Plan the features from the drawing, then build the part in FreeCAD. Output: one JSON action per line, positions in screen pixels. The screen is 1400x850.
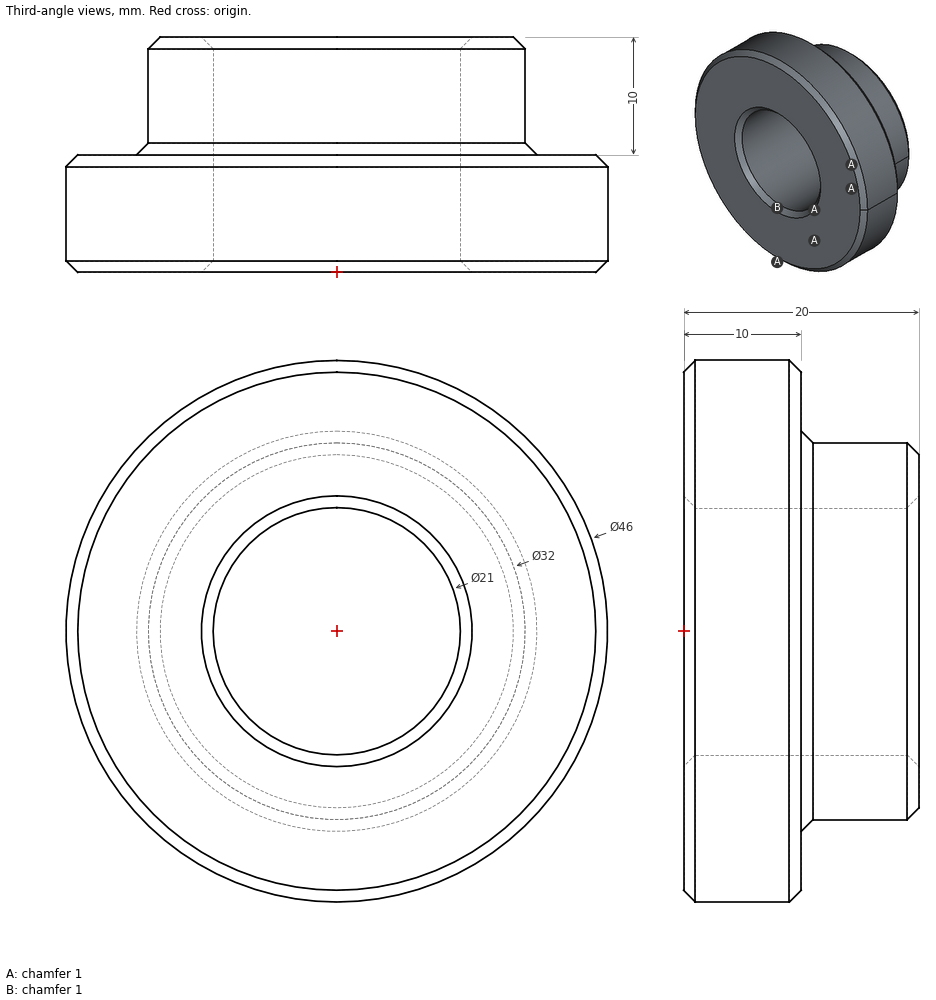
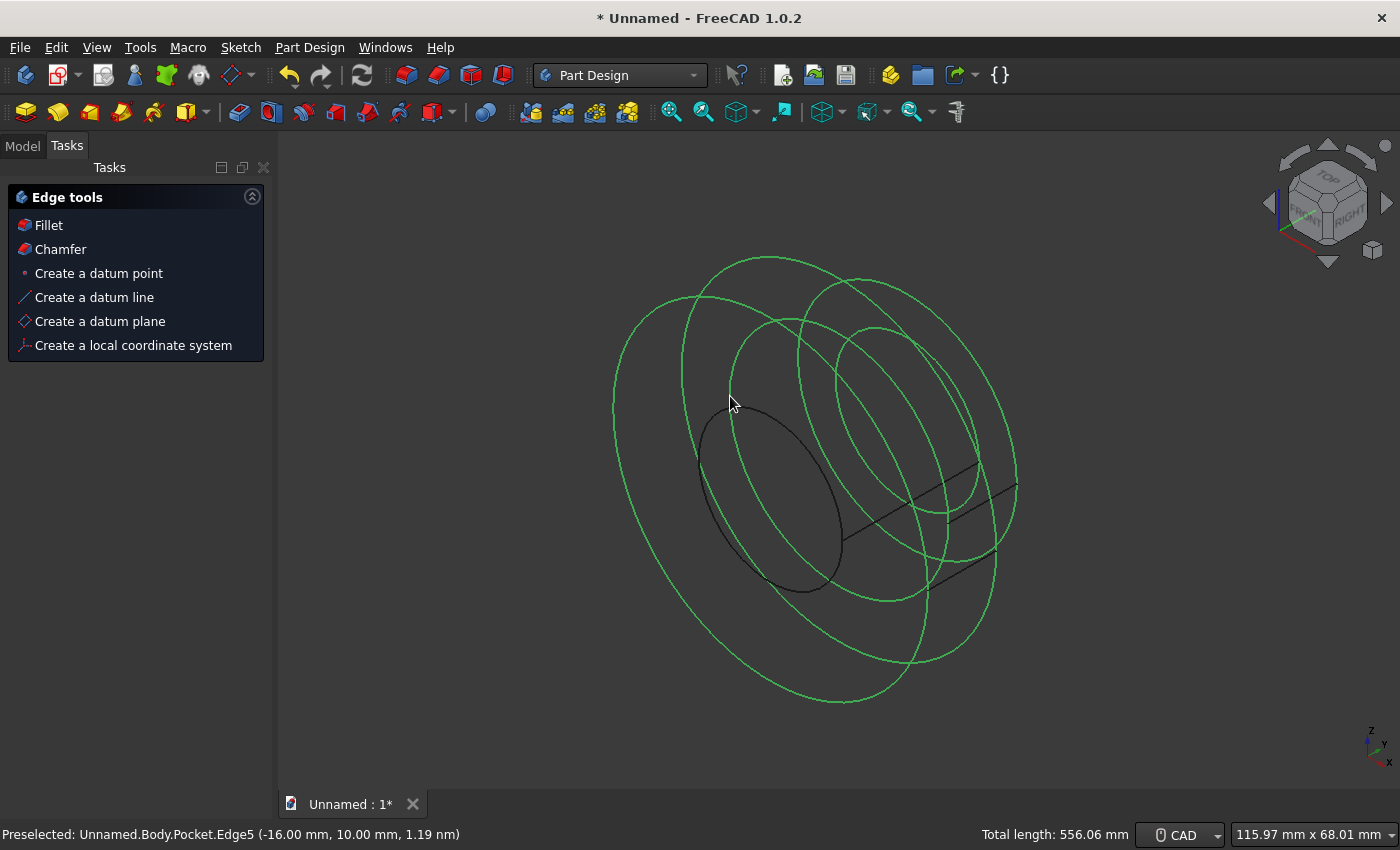
{"action": "key", "text": "v 1"}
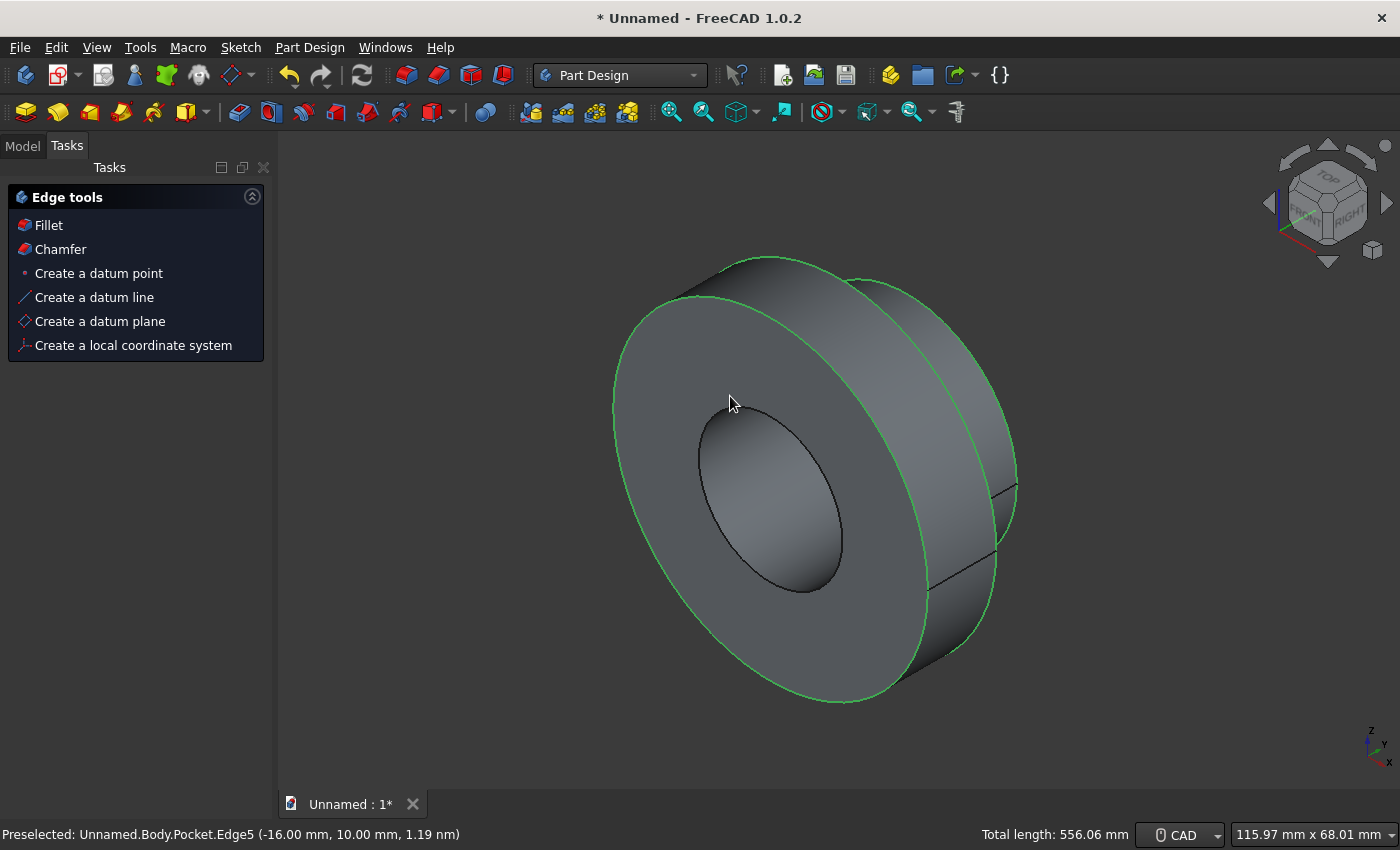
{"action": "left_click", "coordinate": [440, 76]}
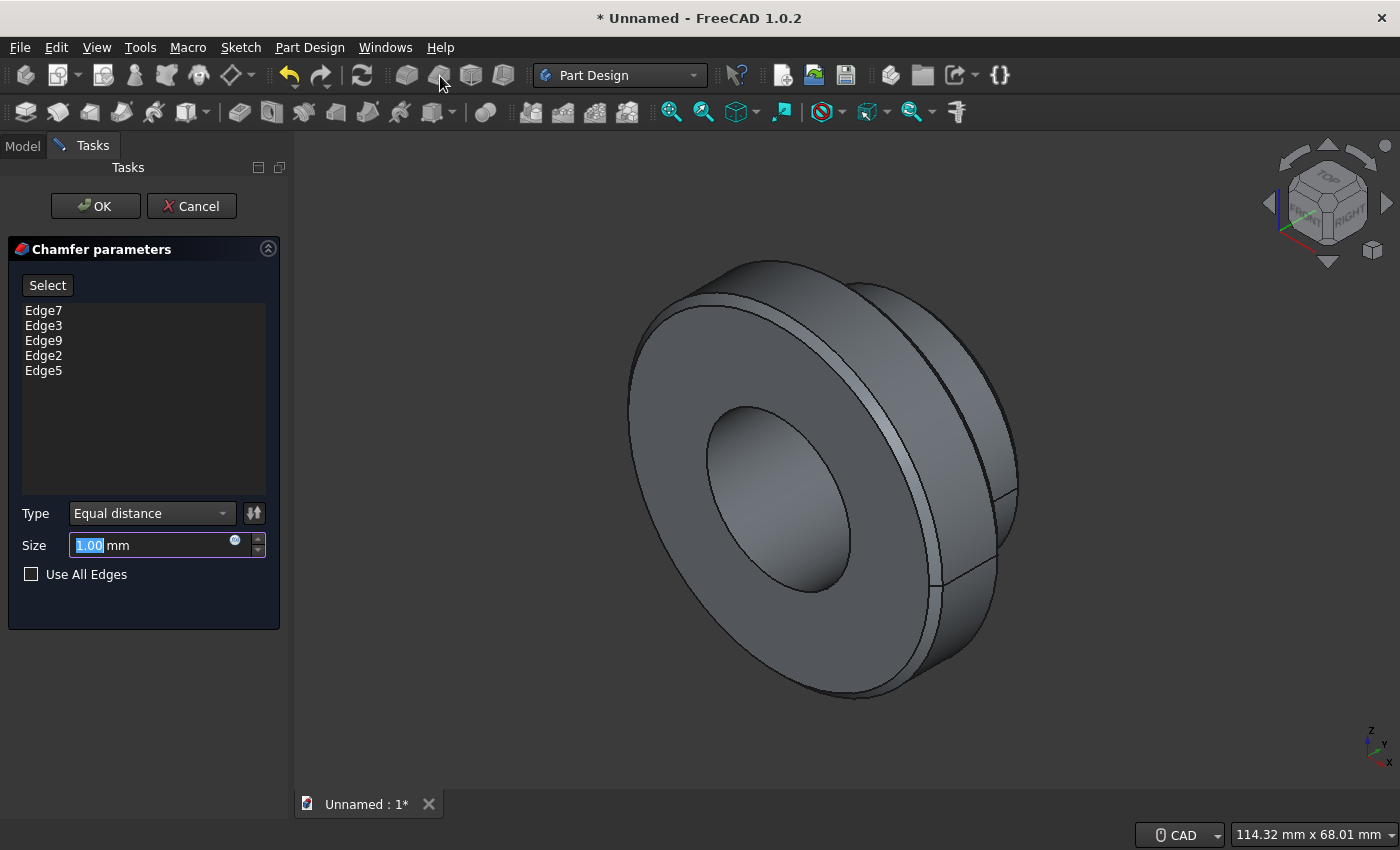
{"action": "type", "text": "1"}
{"action": "key", "text": "Tab"}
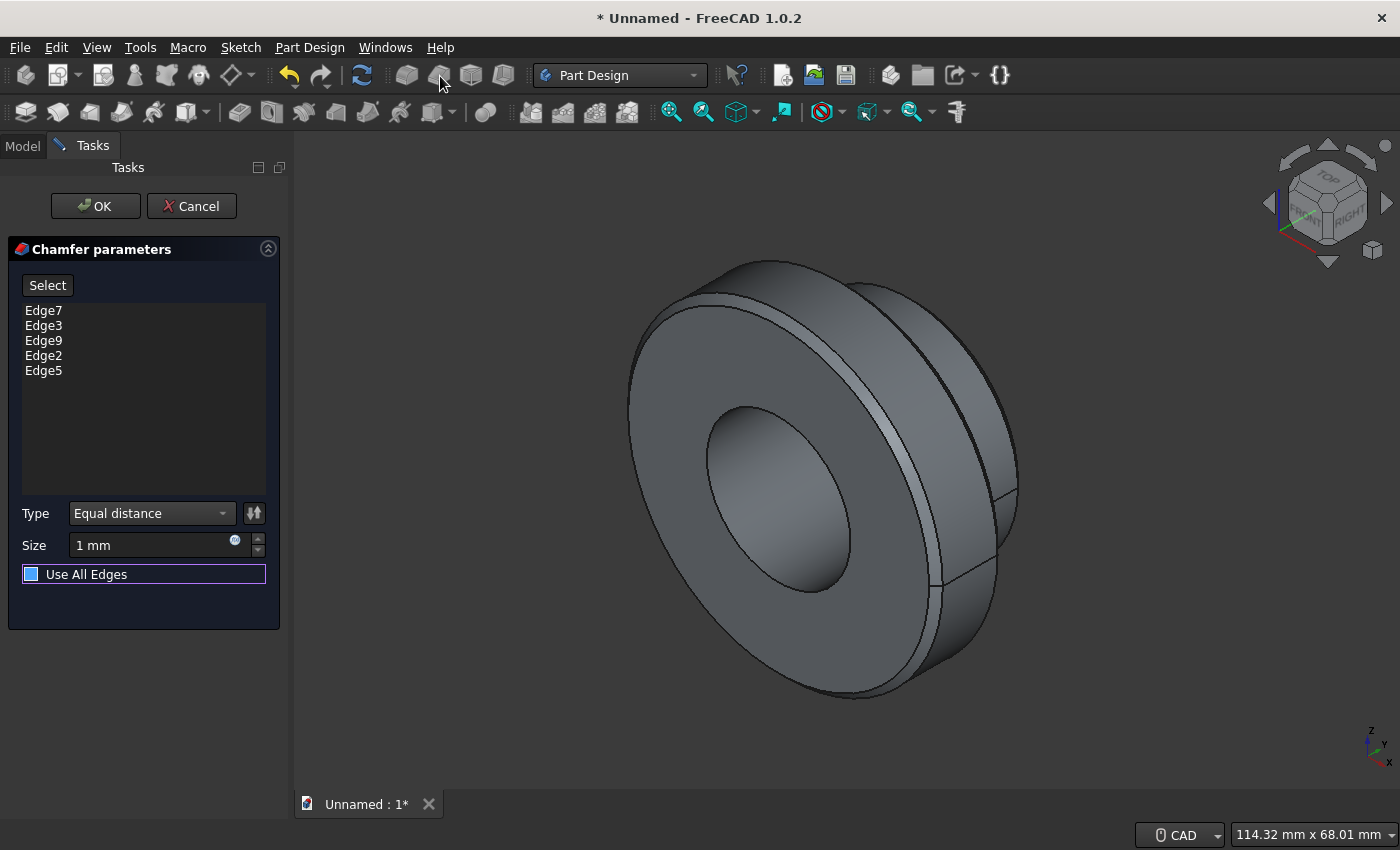
{"action": "left_click", "coordinate": [96, 206]}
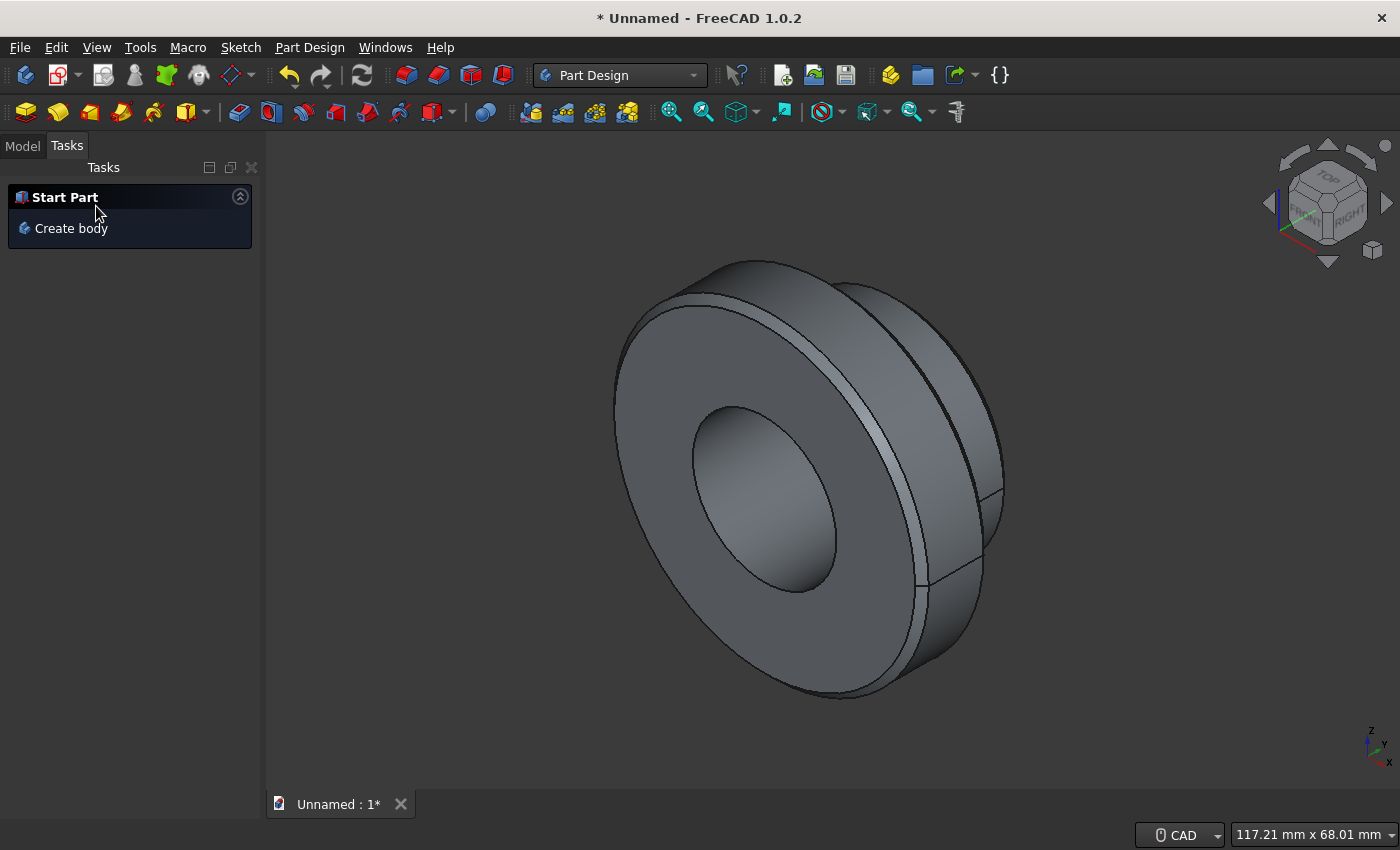
{"action": "left_click", "coordinate": [693, 457]}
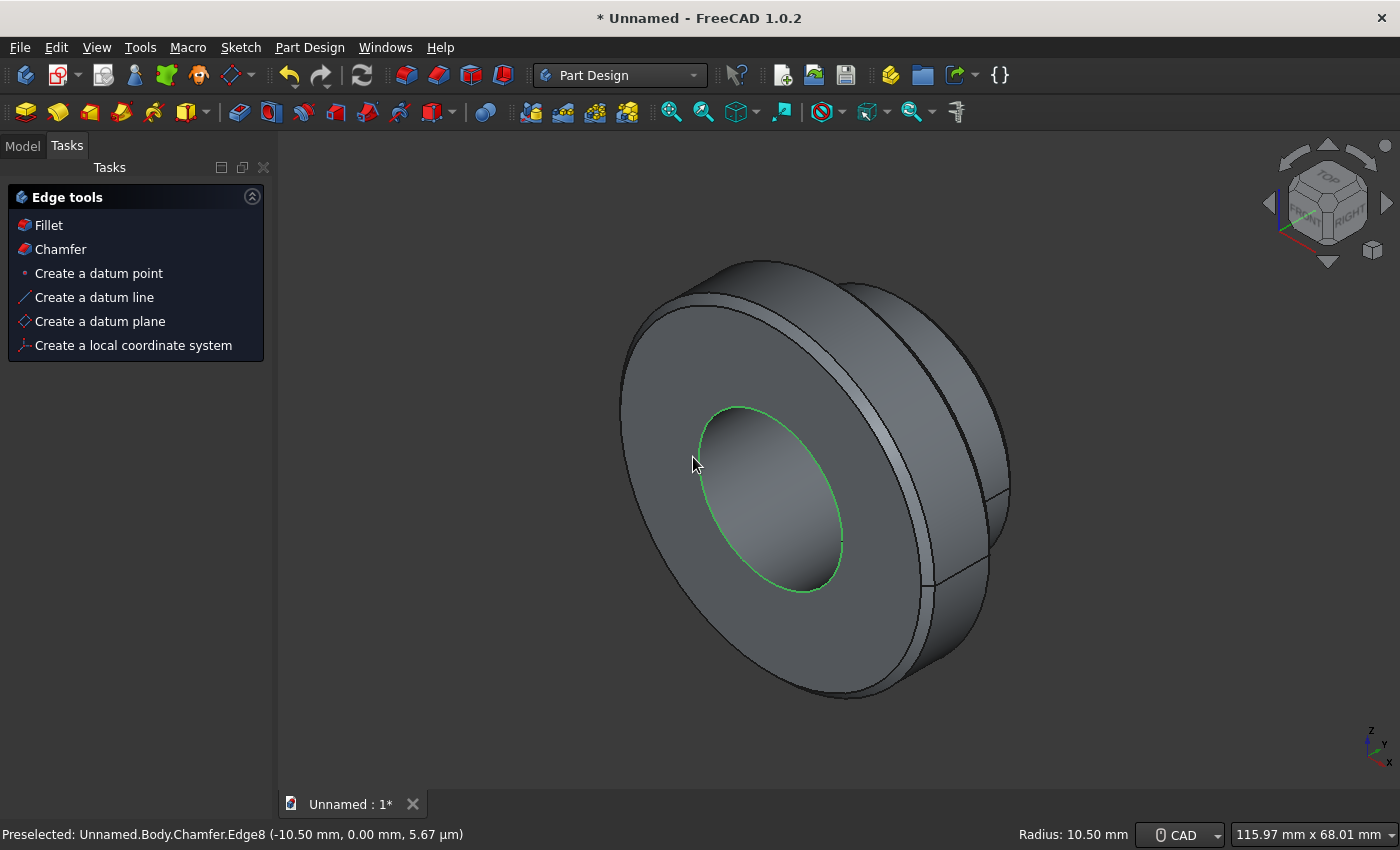
{"action": "left_click", "coordinate": [440, 76]}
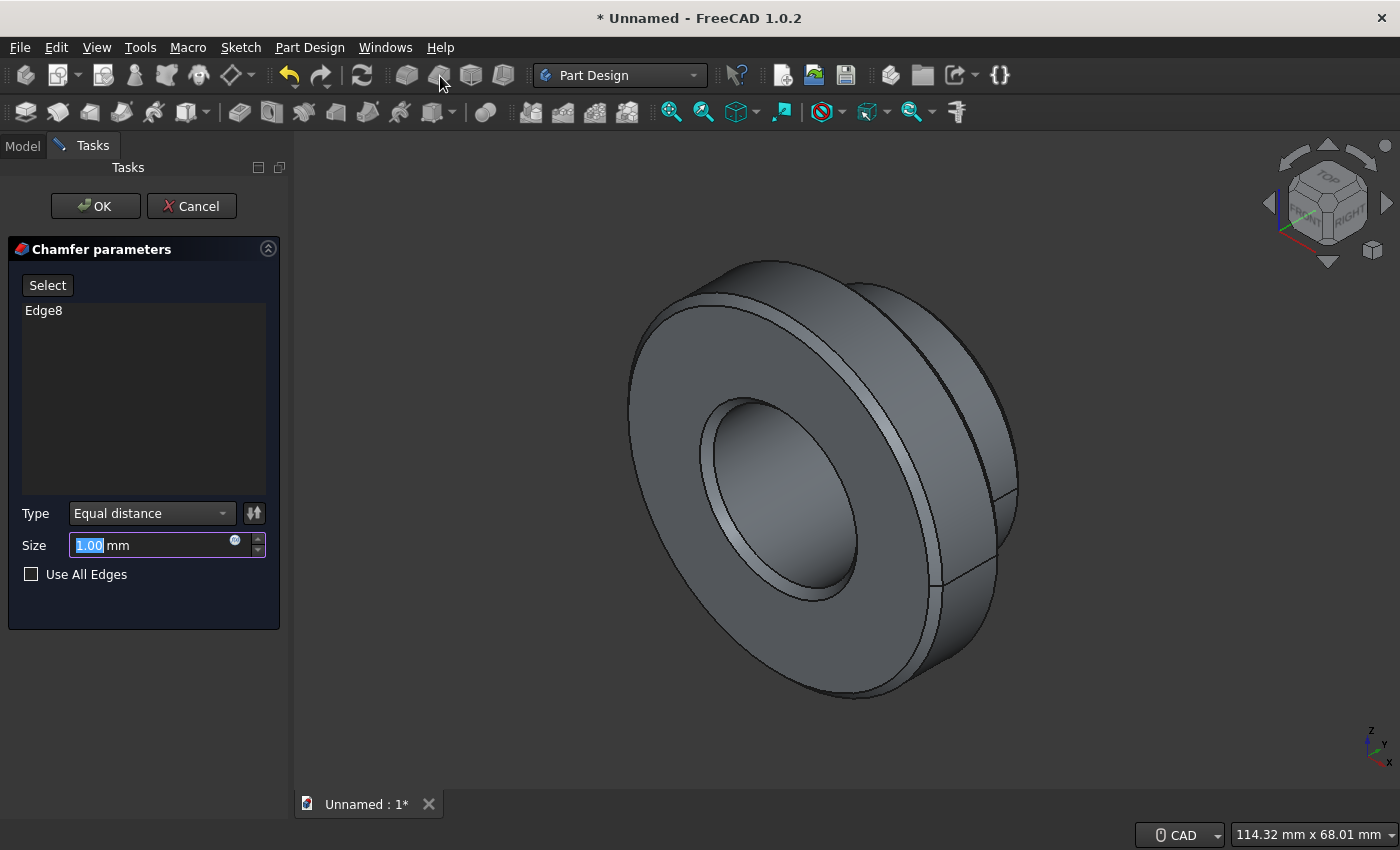
{"action": "type", "text": "1"}
{"action": "key", "text": "Tab"}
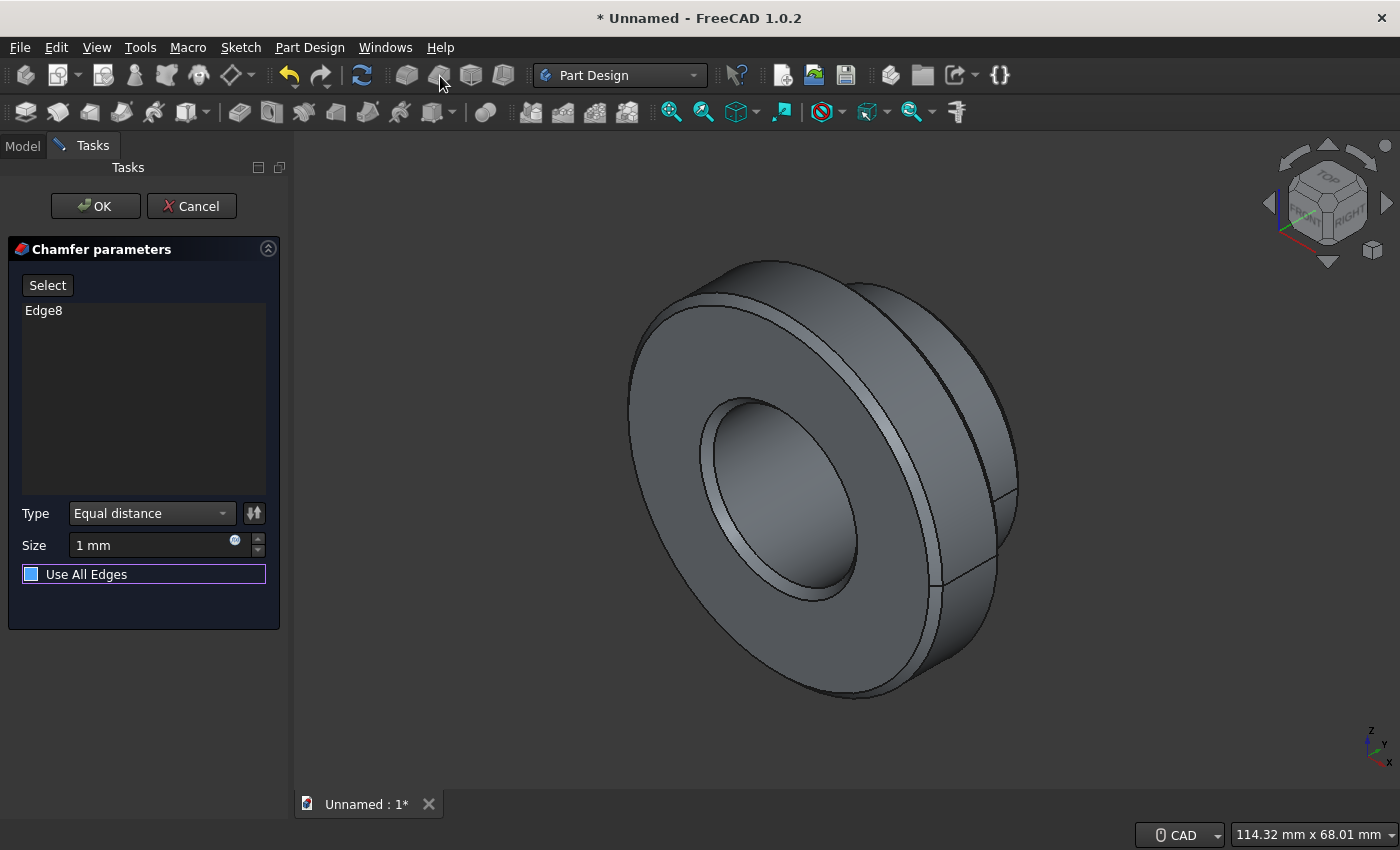
{"action": "left_click", "coordinate": [96, 206]}